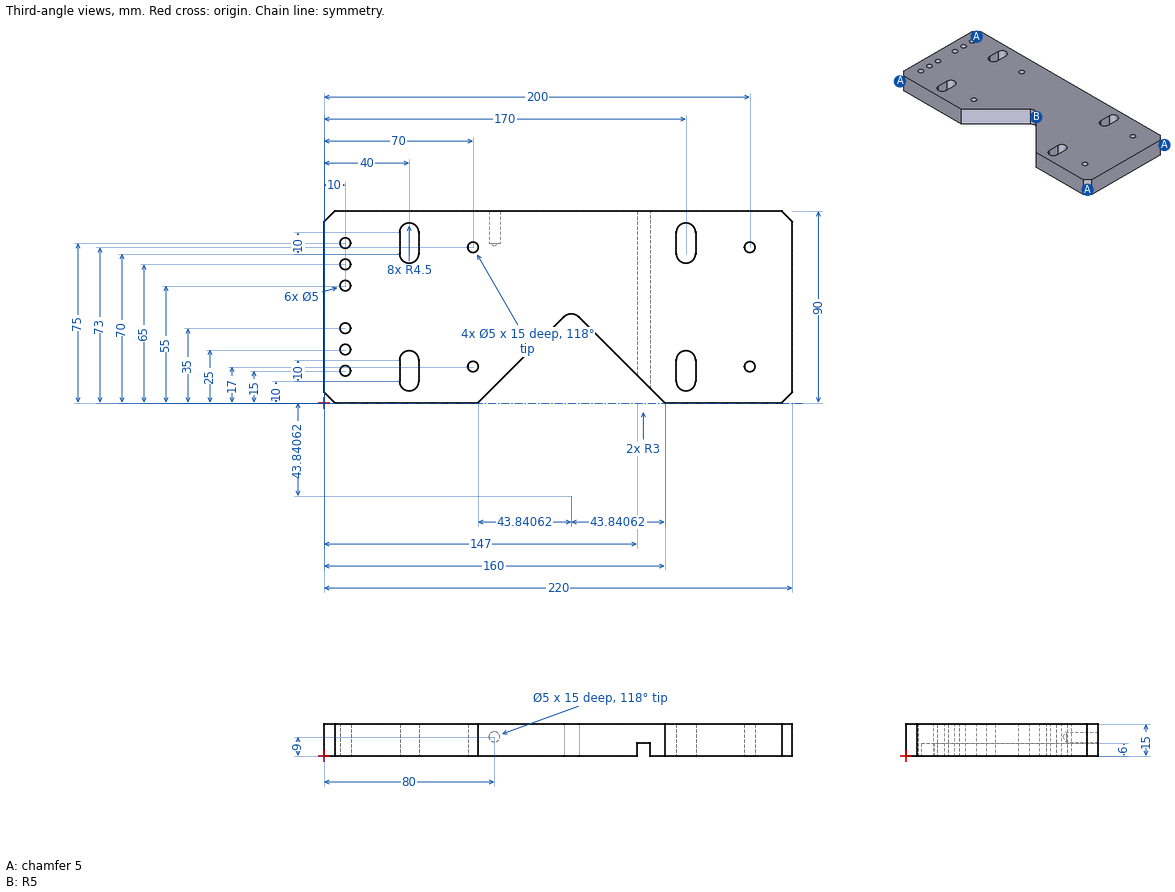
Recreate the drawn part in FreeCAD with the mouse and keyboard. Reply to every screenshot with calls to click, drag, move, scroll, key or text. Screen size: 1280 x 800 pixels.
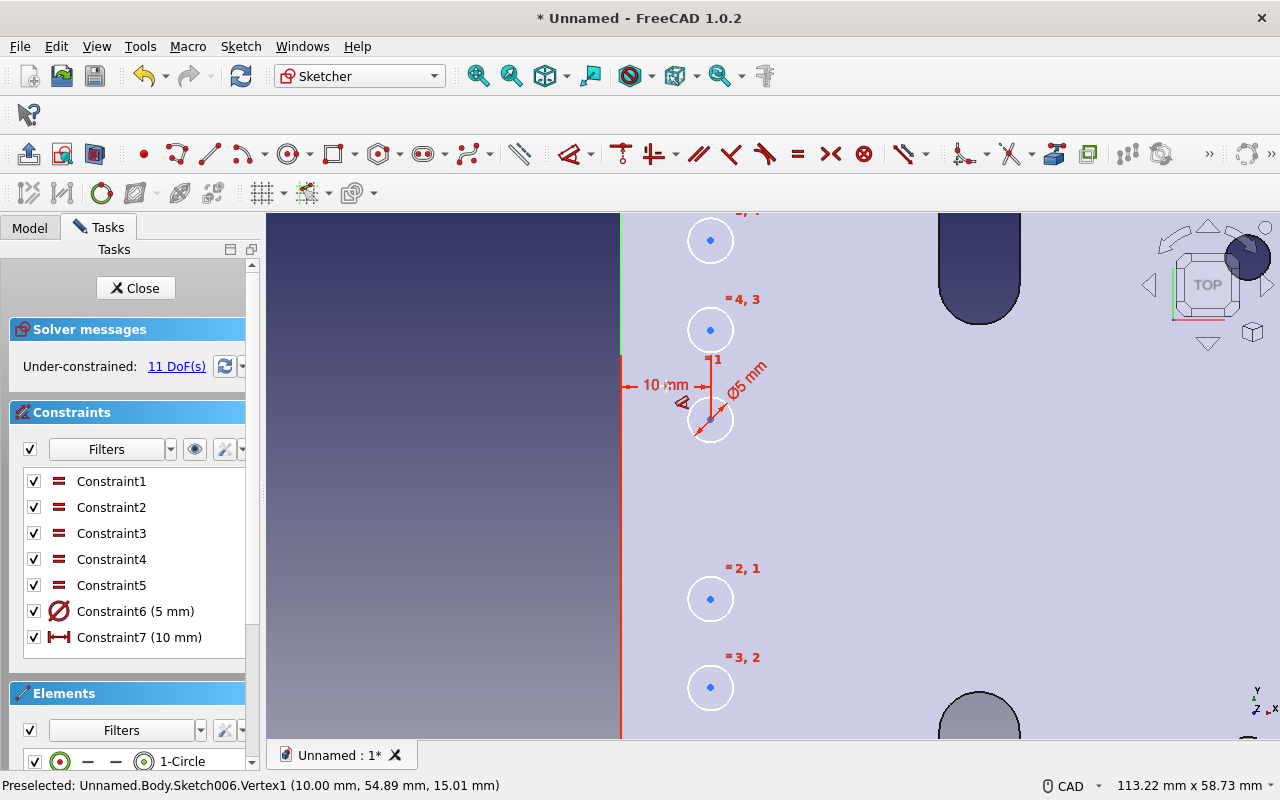
click(711, 420)
click(587, 565)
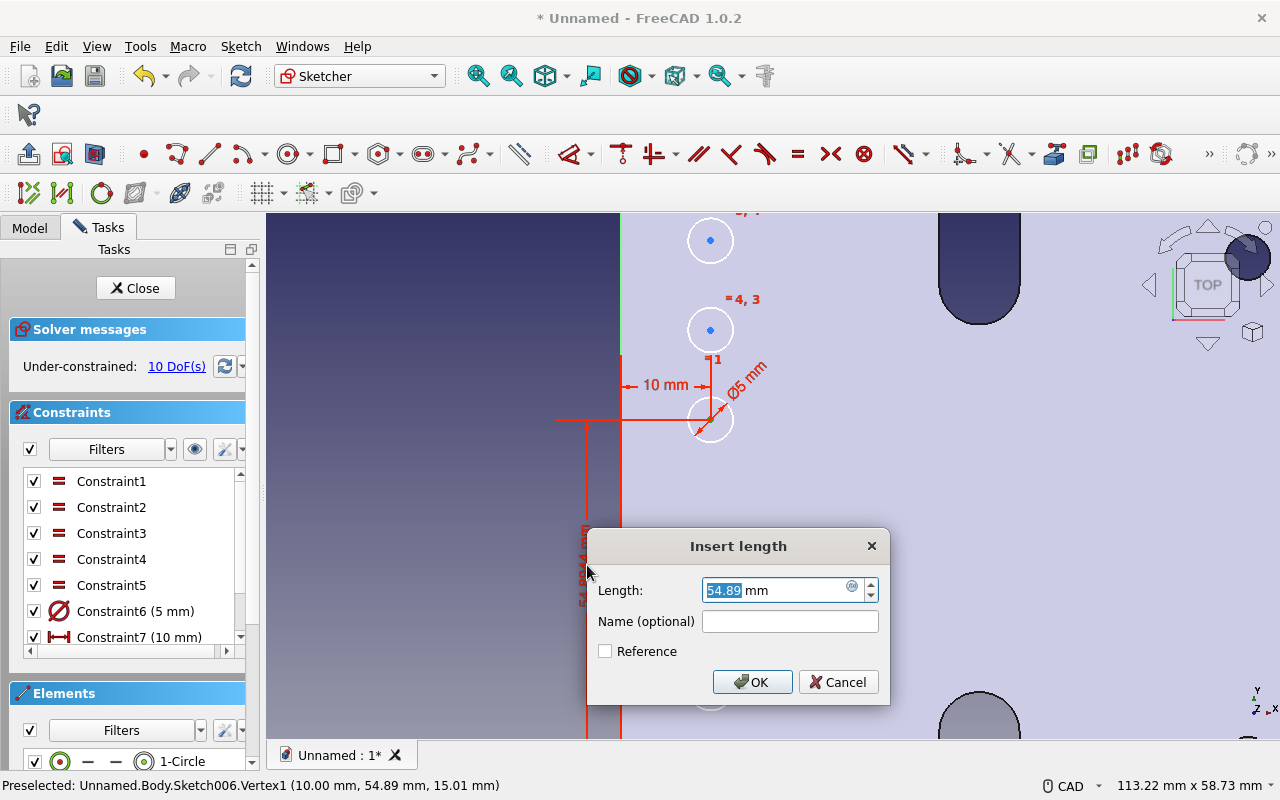
text(55)
key(Return)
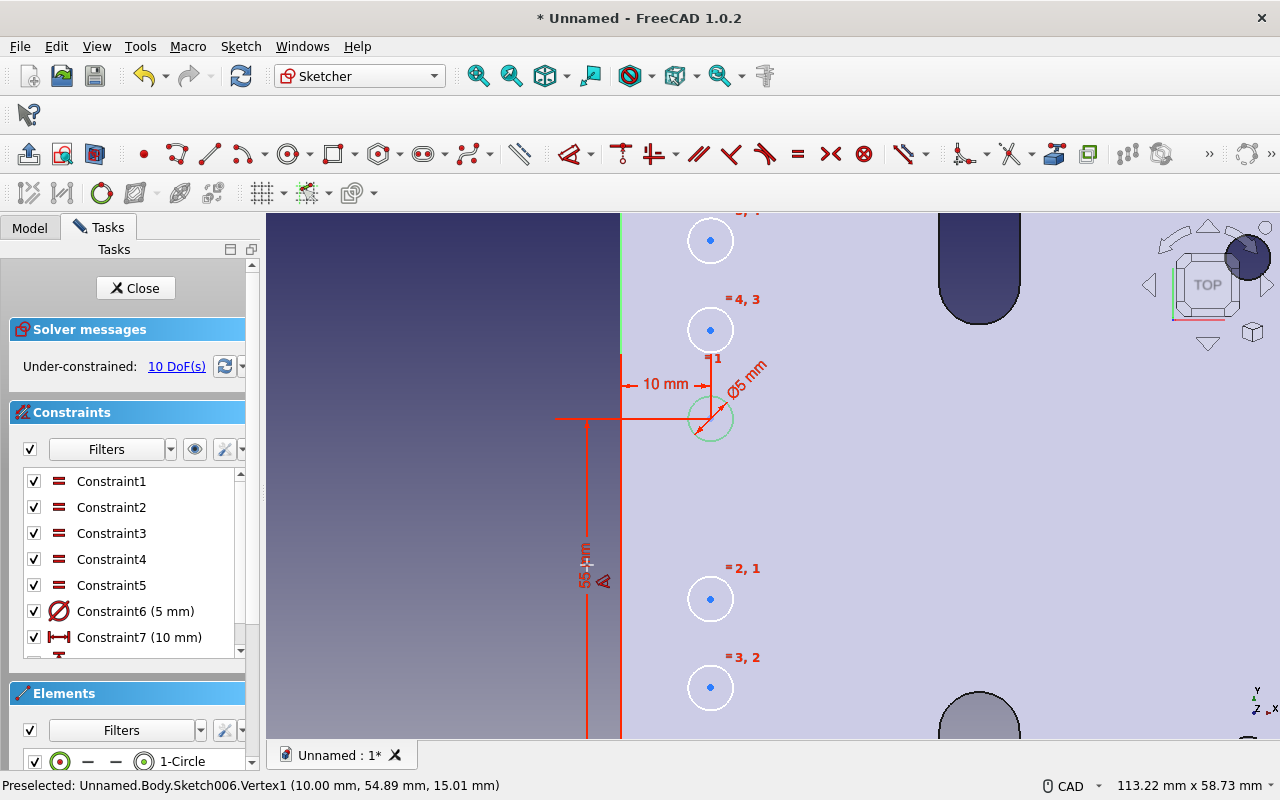
click(711, 599)
click(666, 565)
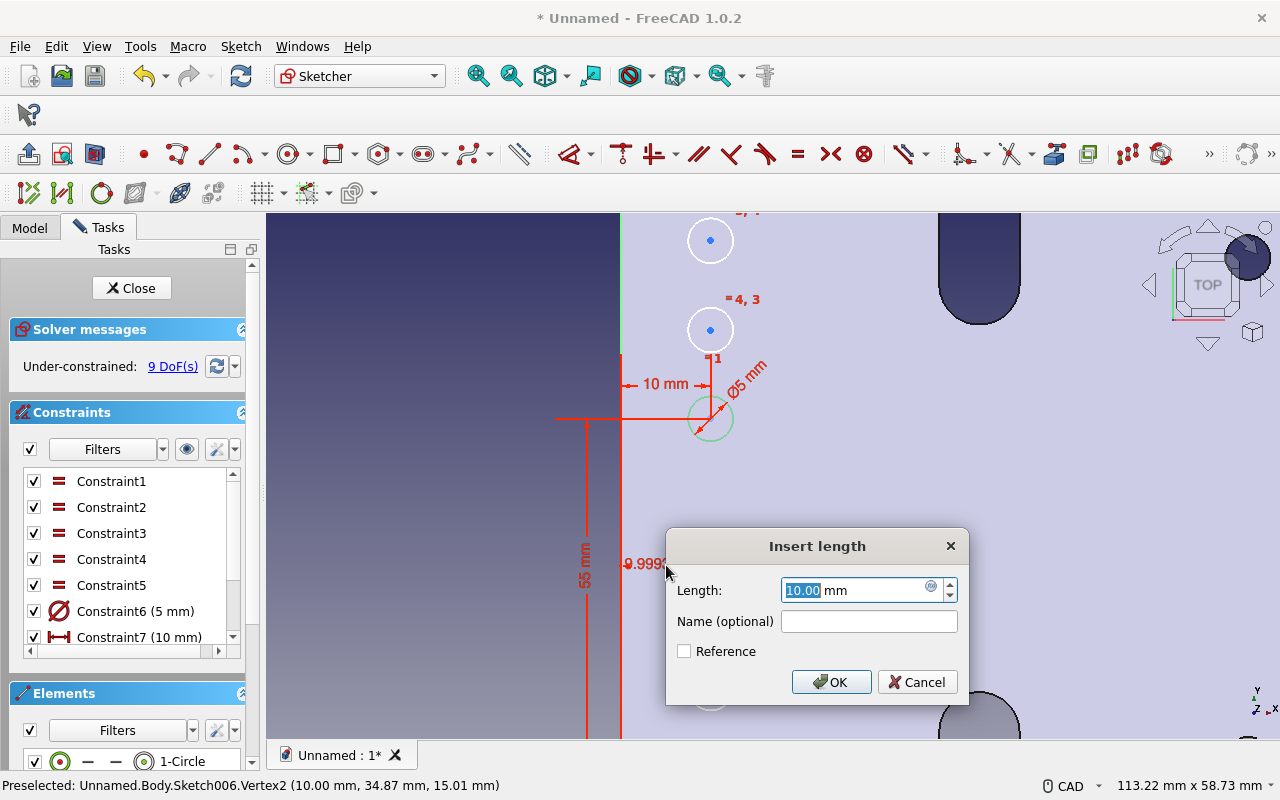
text(10)
key(Return)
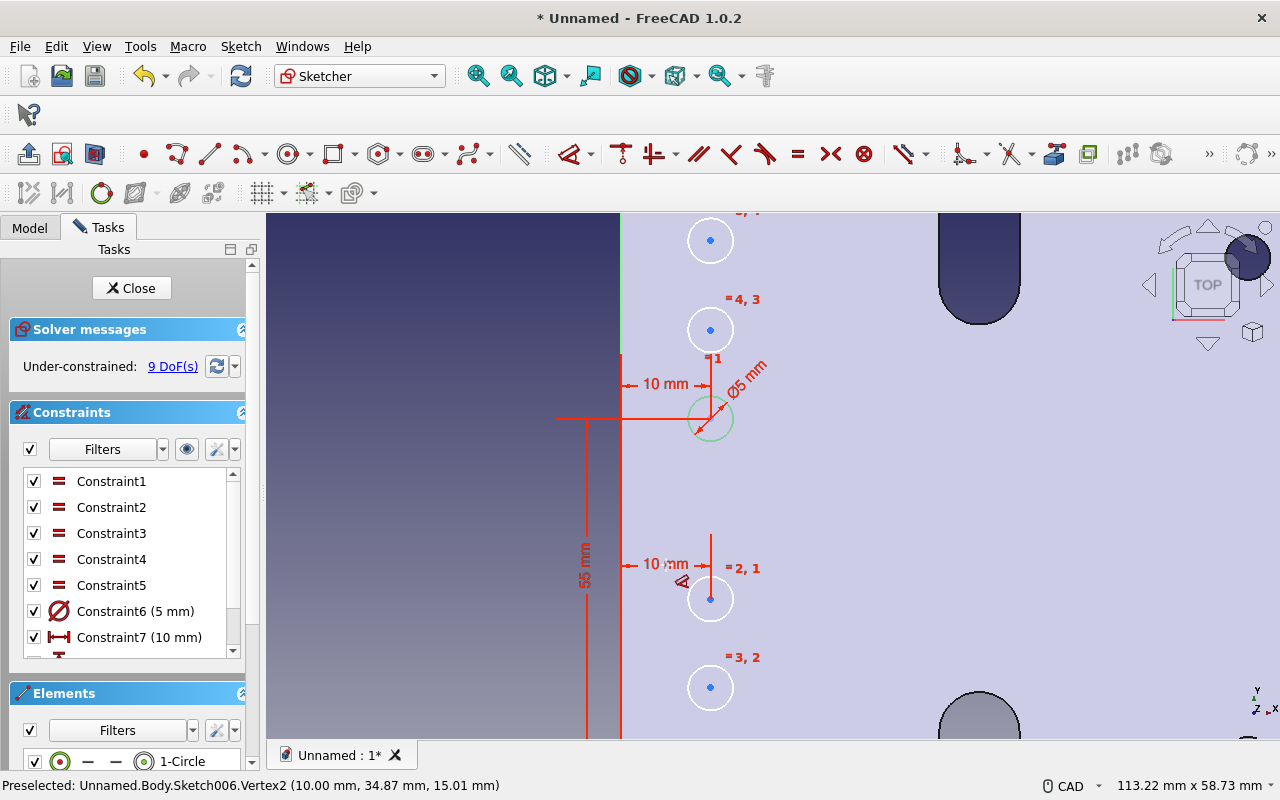
click(711, 599)
click(587, 655)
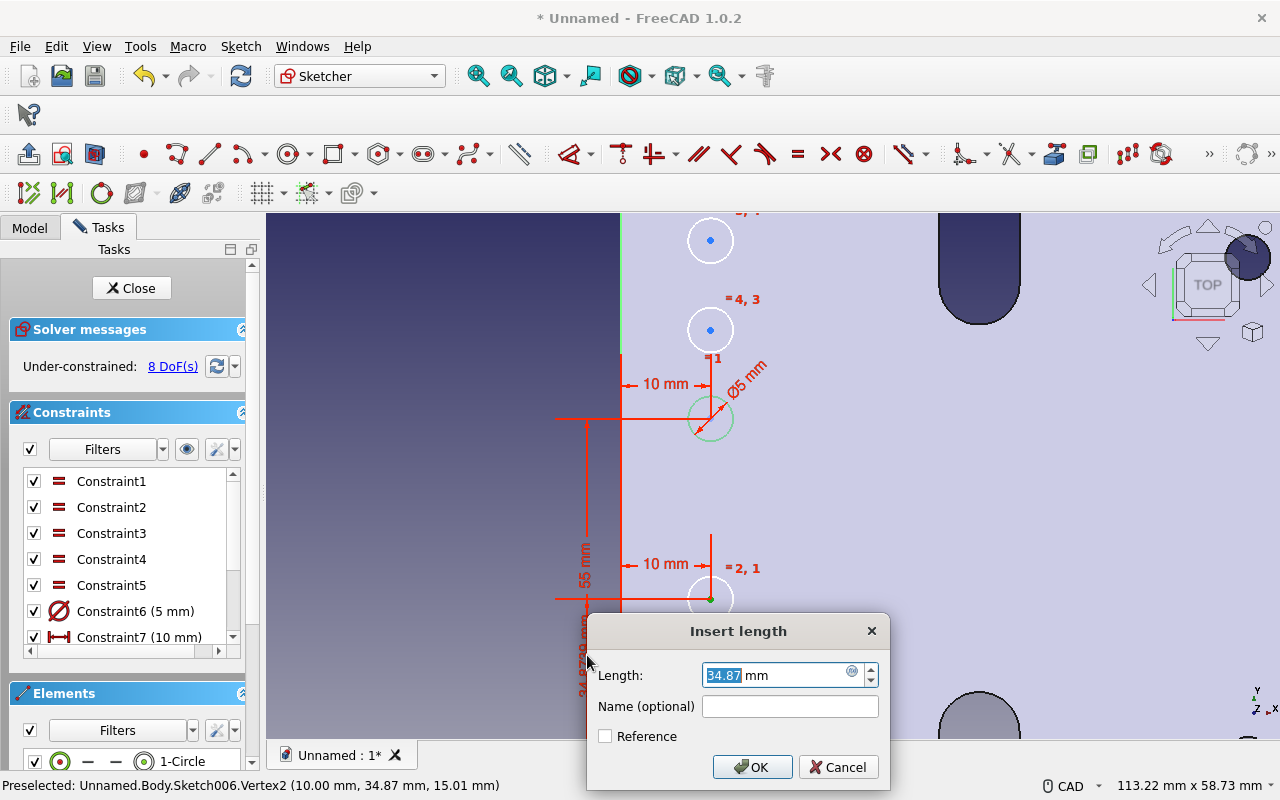
text(35)
key(Return)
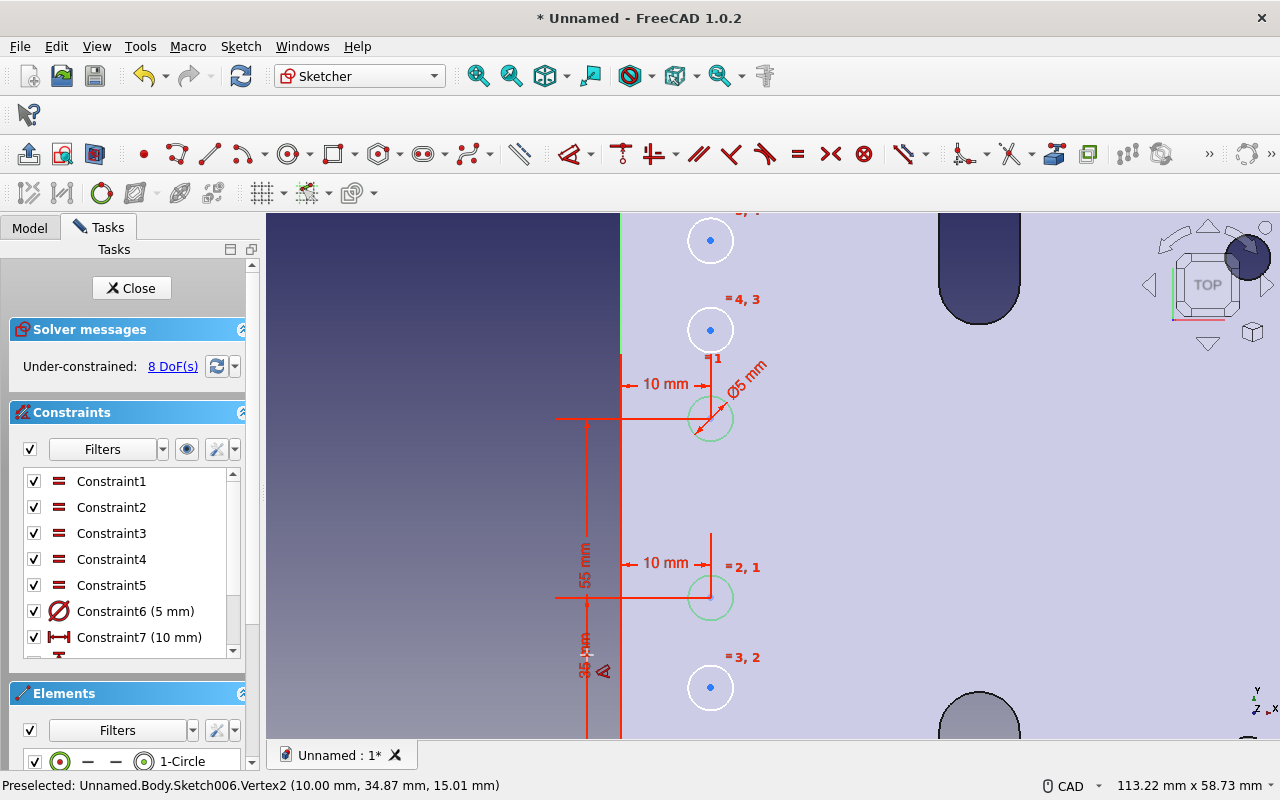
click(711, 688)
click(666, 654)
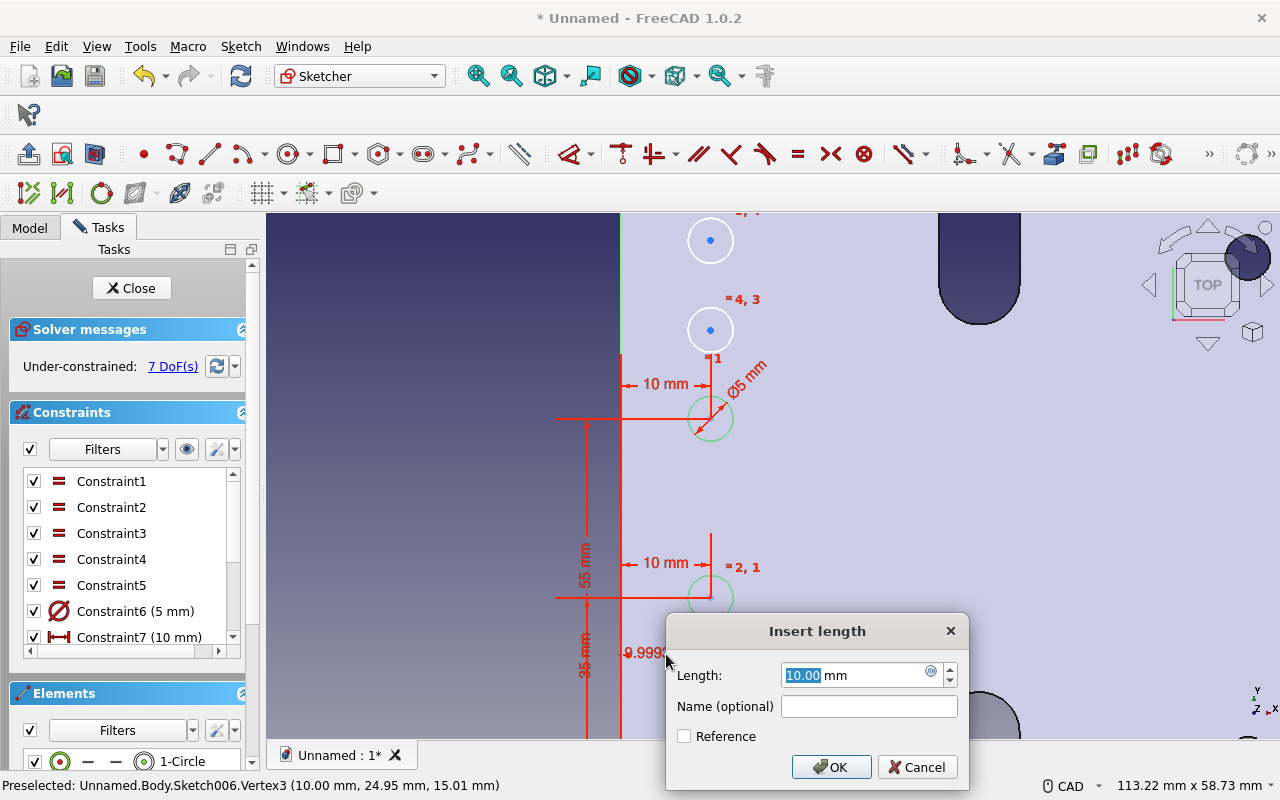
text(10)
key(Return)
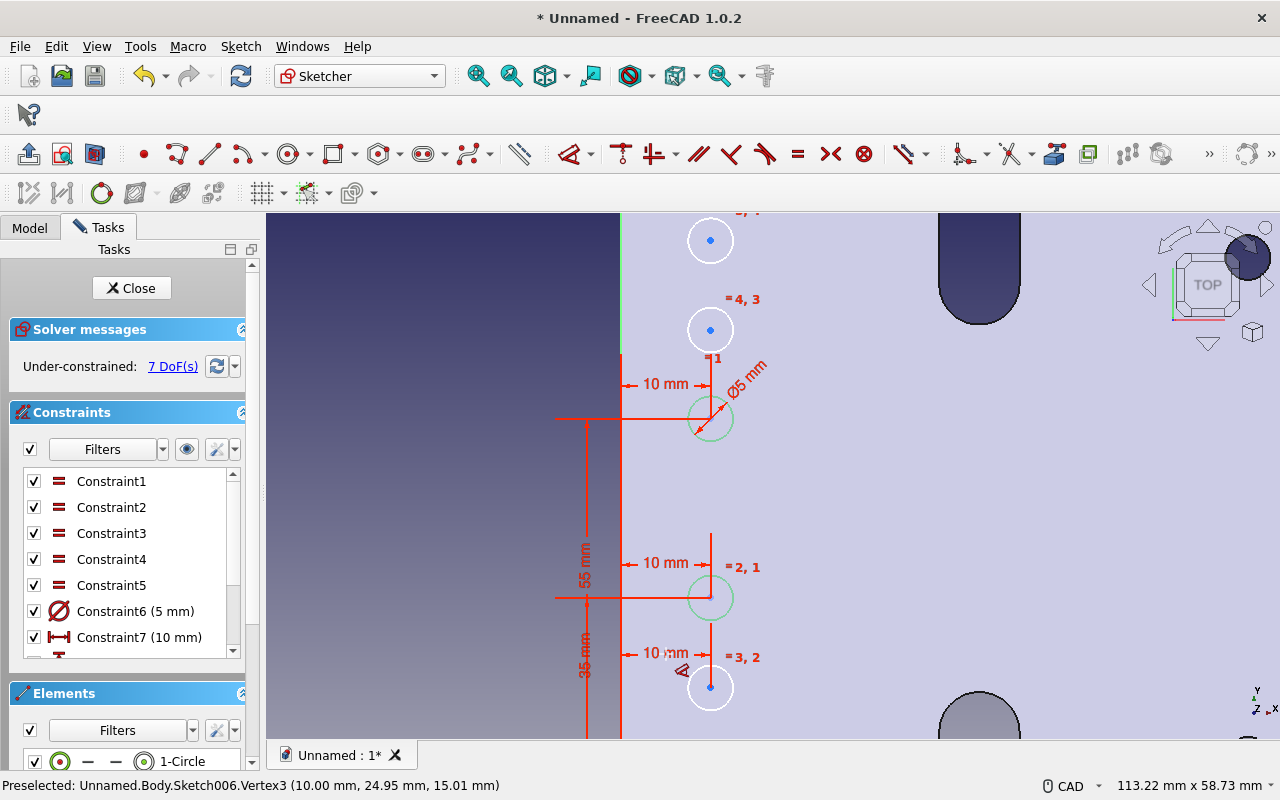
click(711, 688)
click(587, 699)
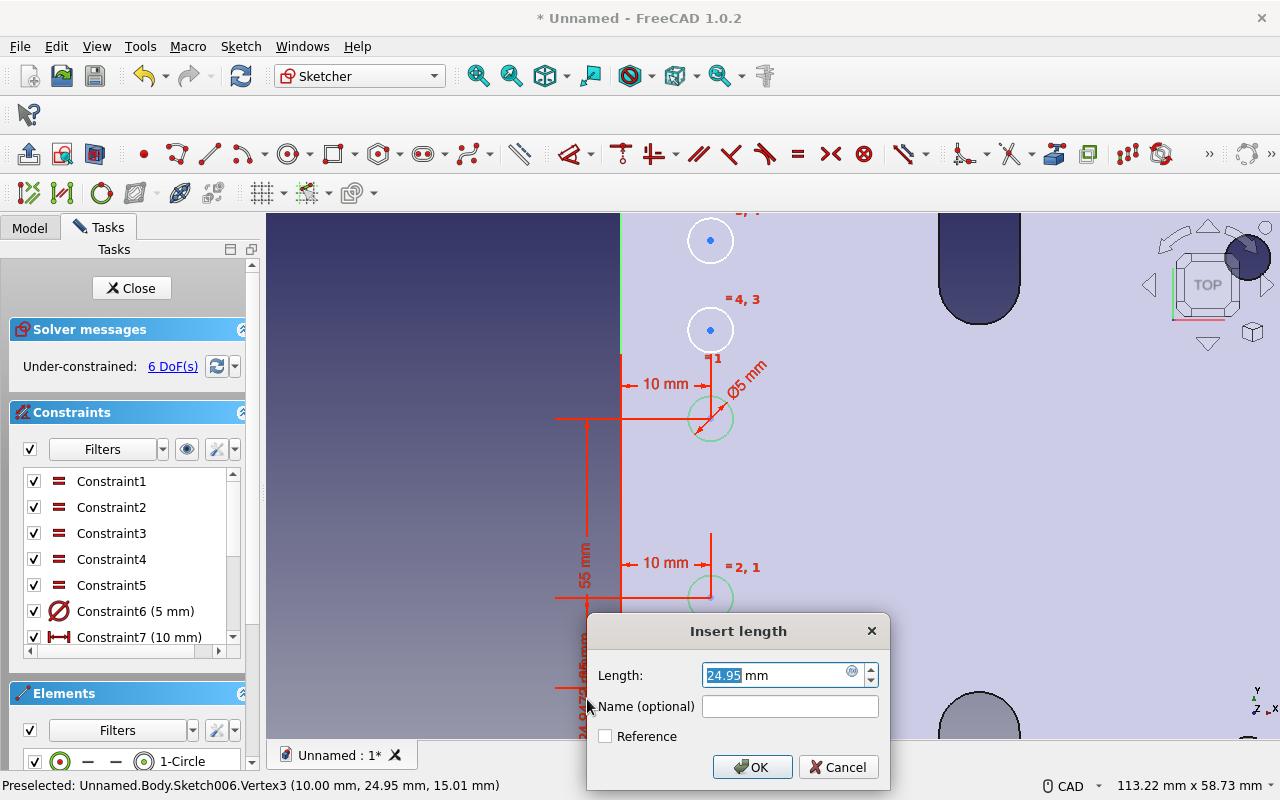
text(25)
key(Return)